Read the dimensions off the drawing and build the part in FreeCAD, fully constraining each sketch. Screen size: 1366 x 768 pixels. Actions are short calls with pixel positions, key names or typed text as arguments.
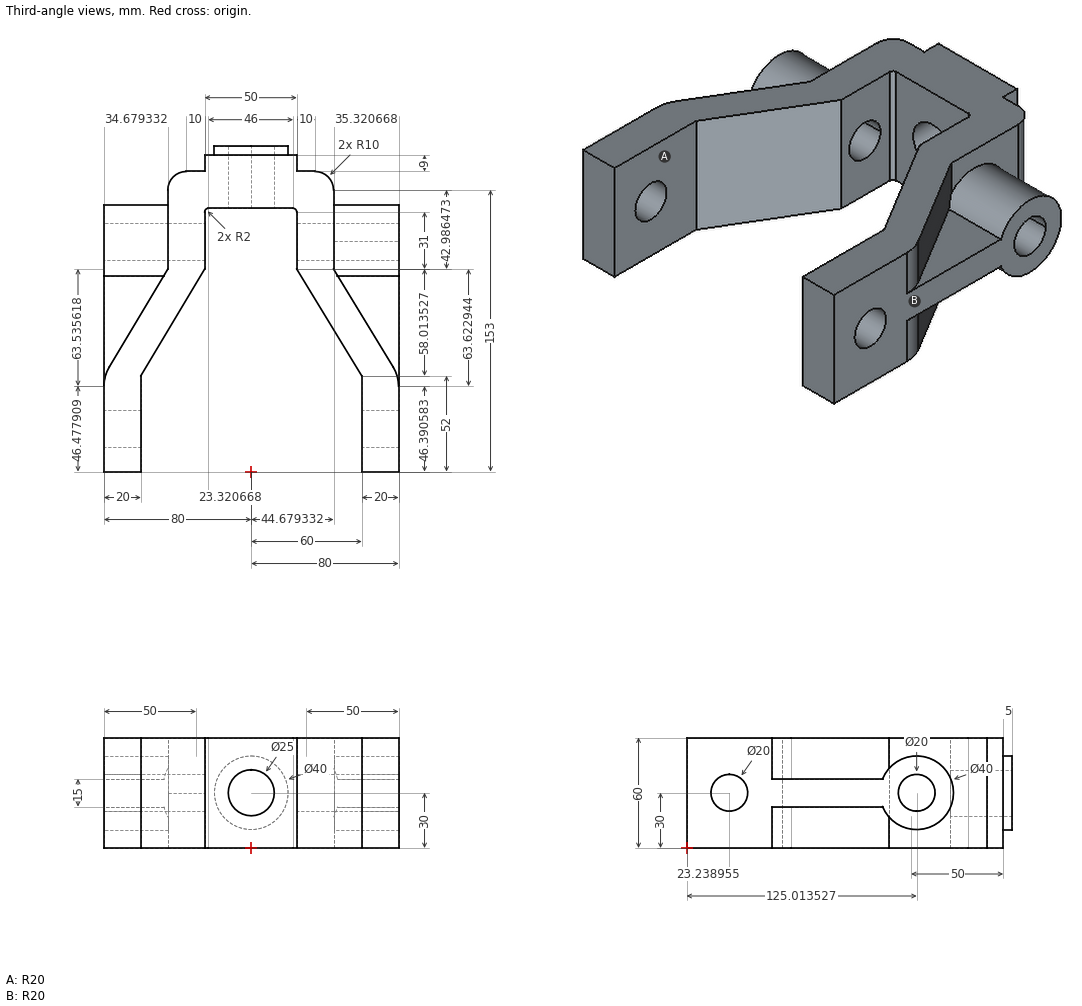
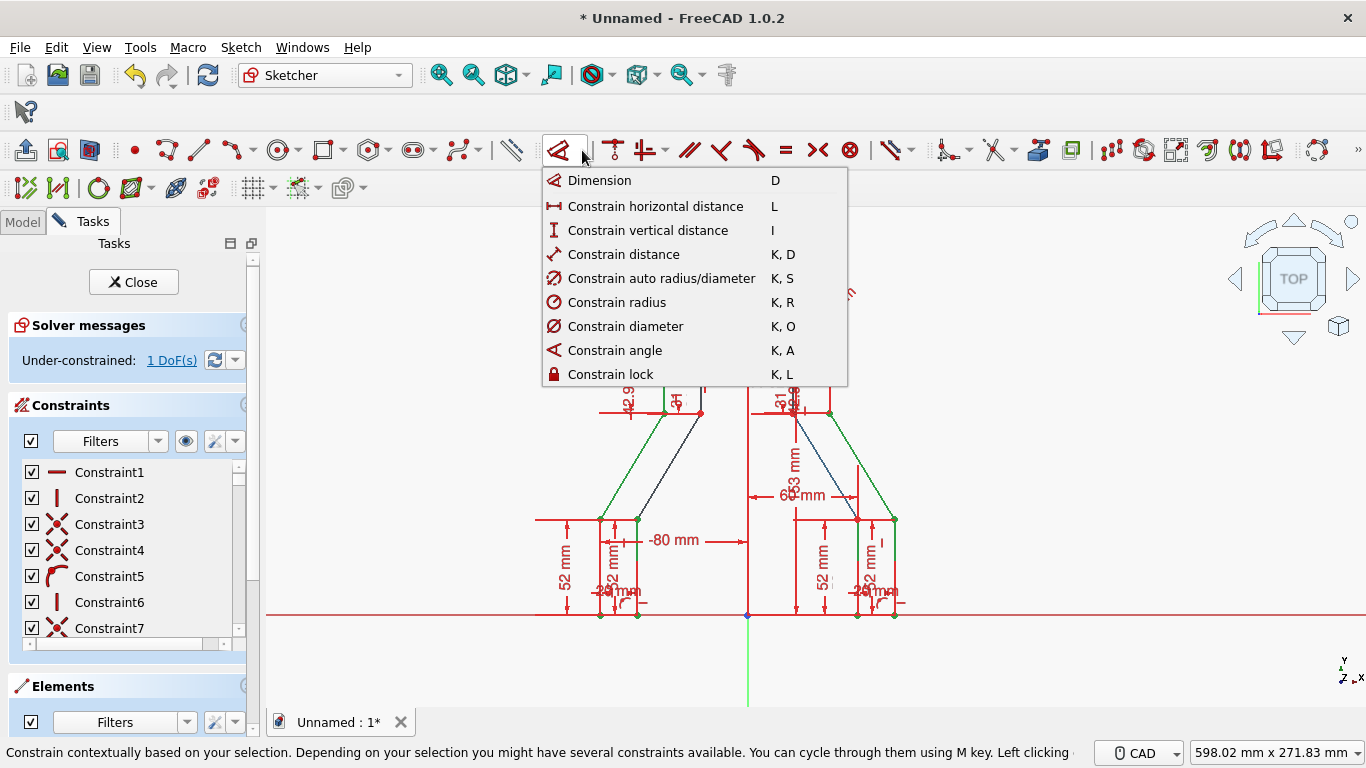
click(695, 230)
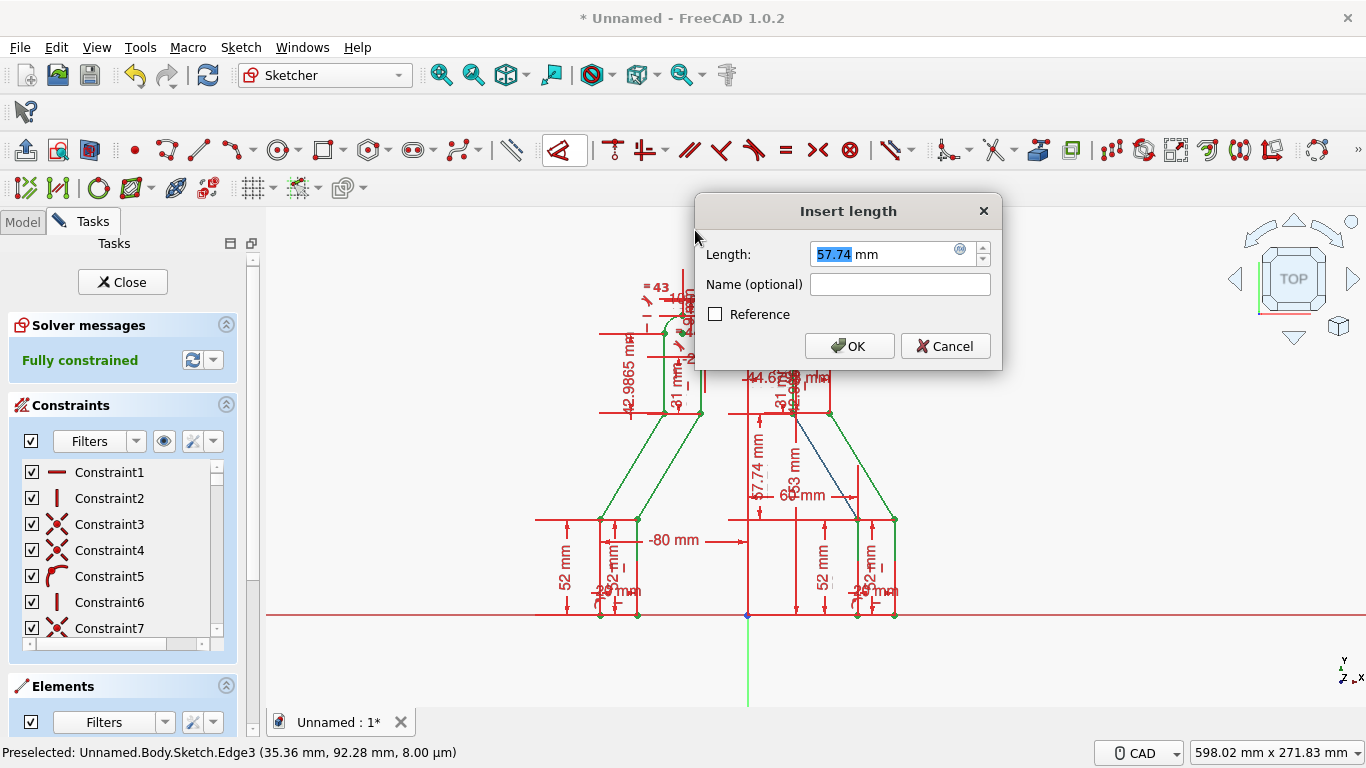
text(58.013527)
key(Return)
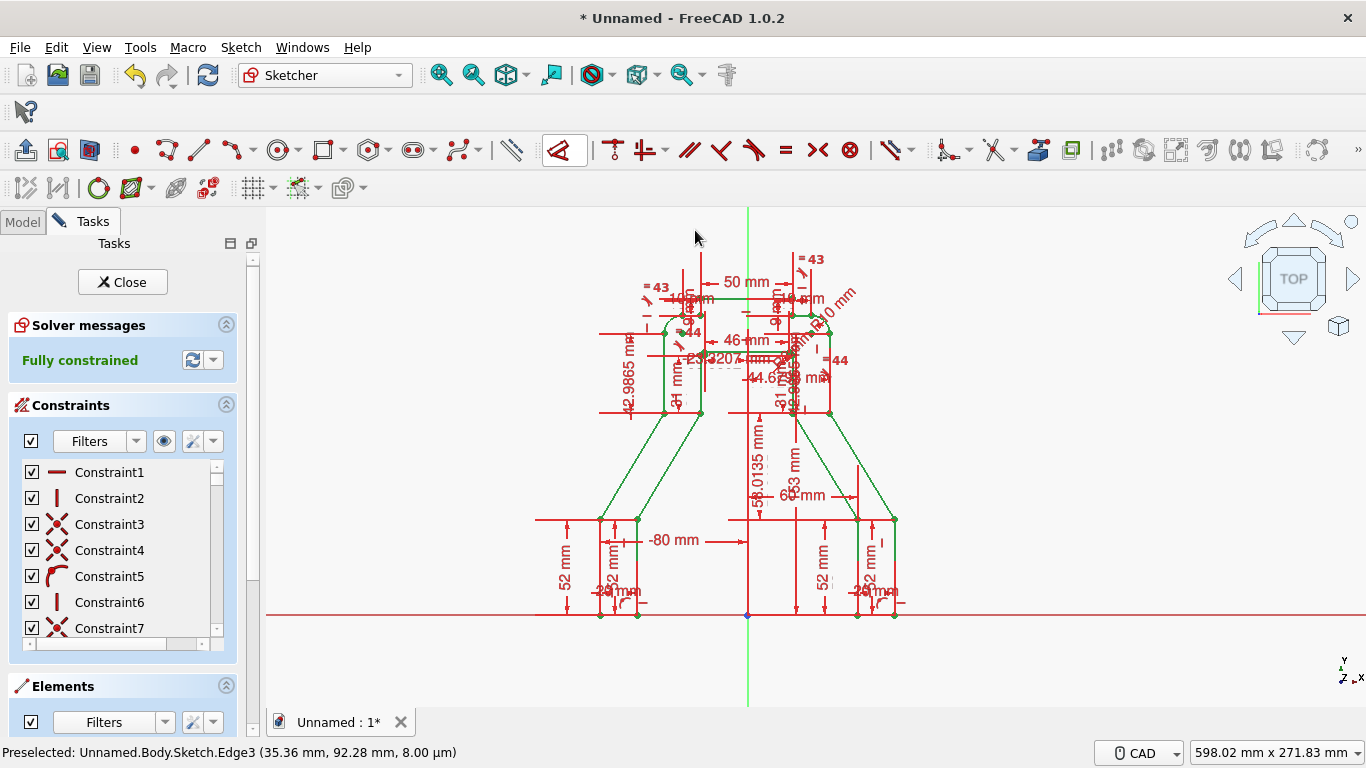
click(123, 282)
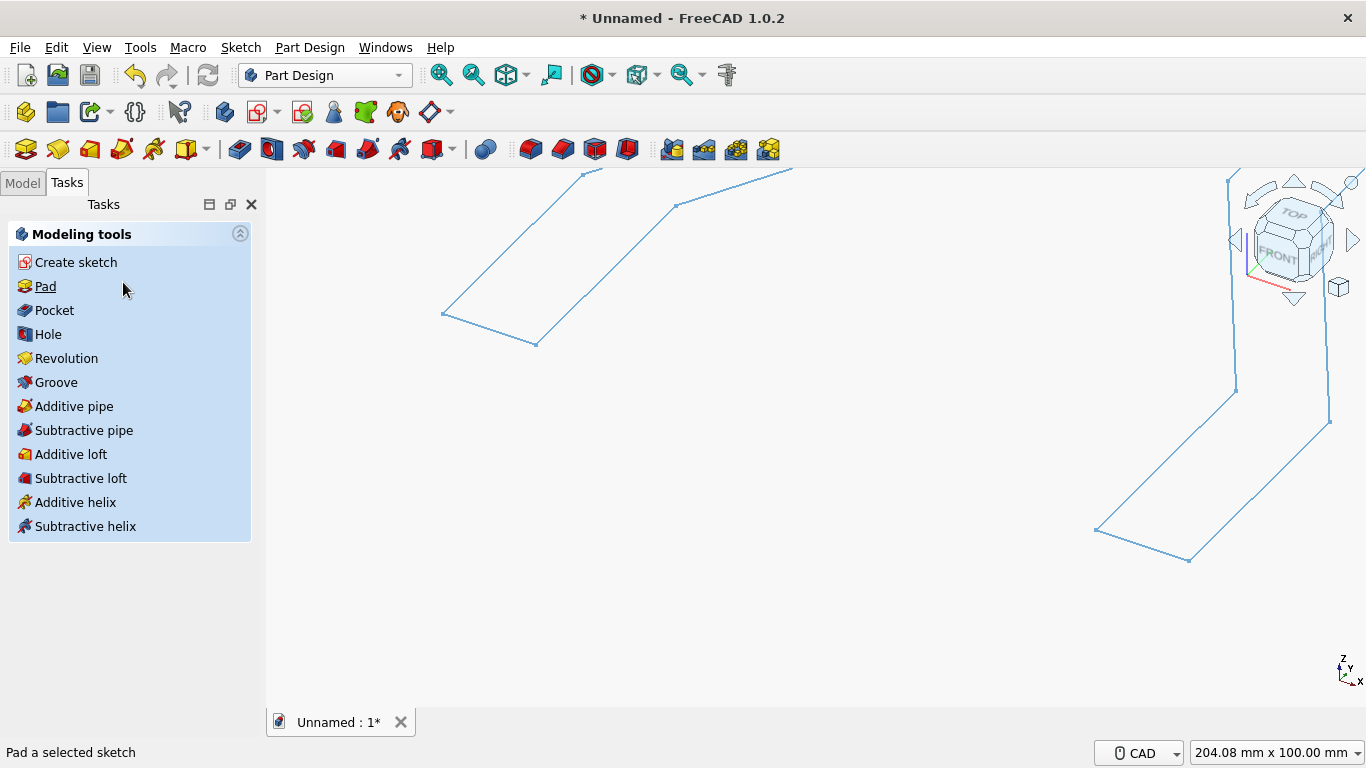
click(26, 150)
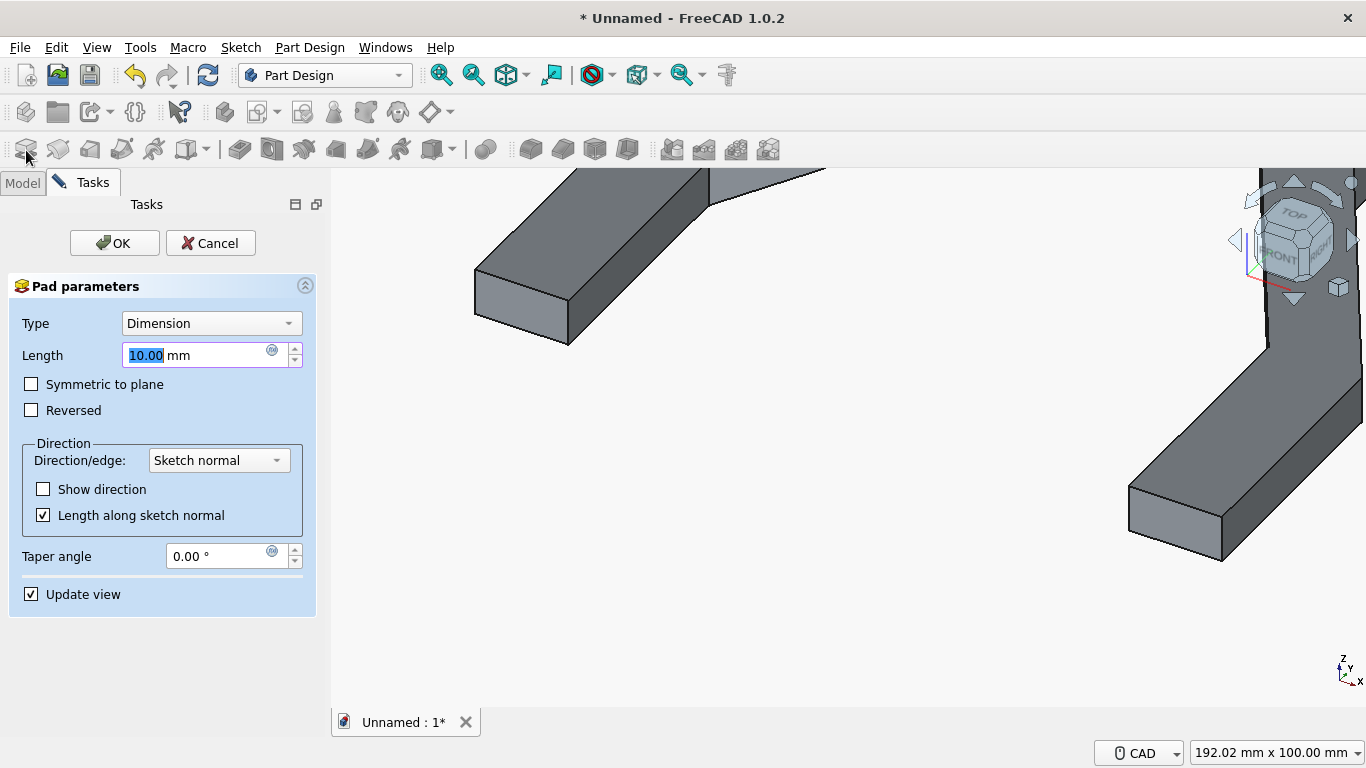
text(60)
key(Tab)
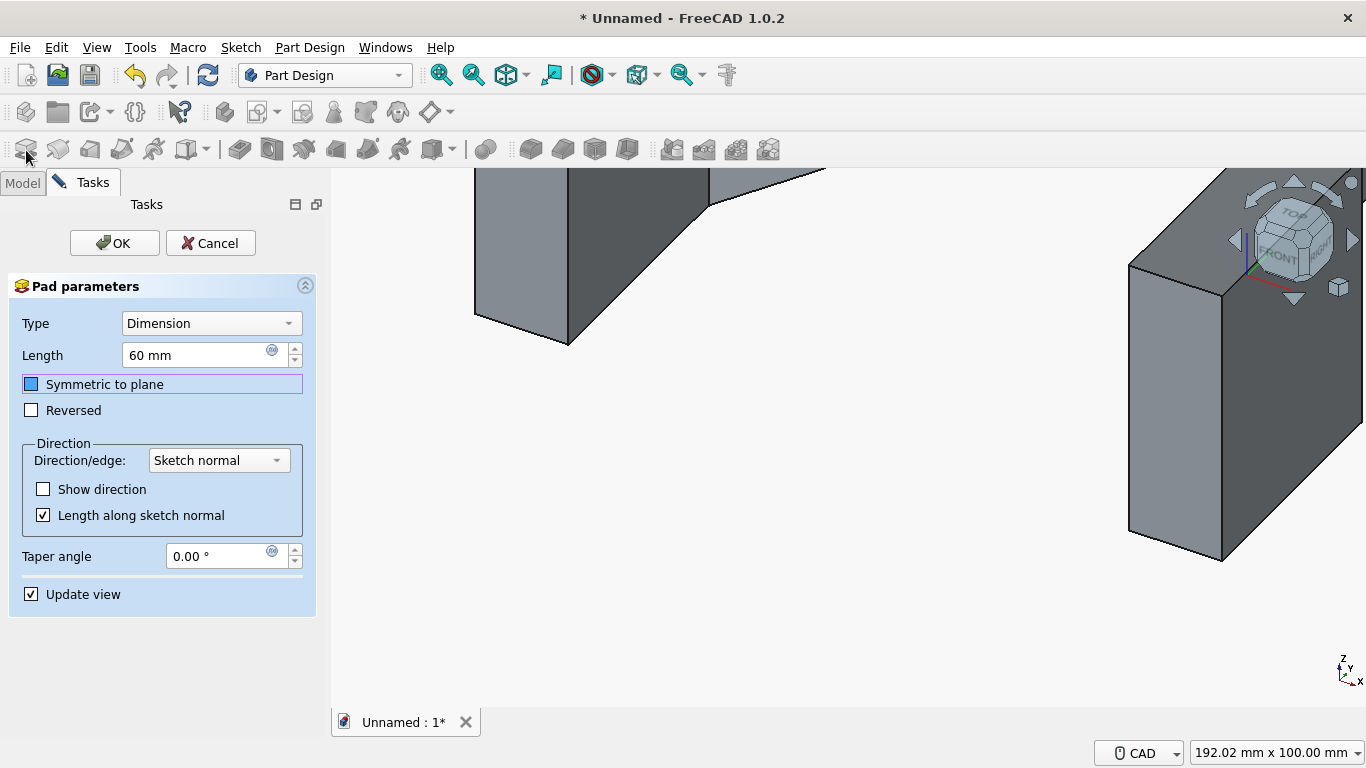
click(115, 243)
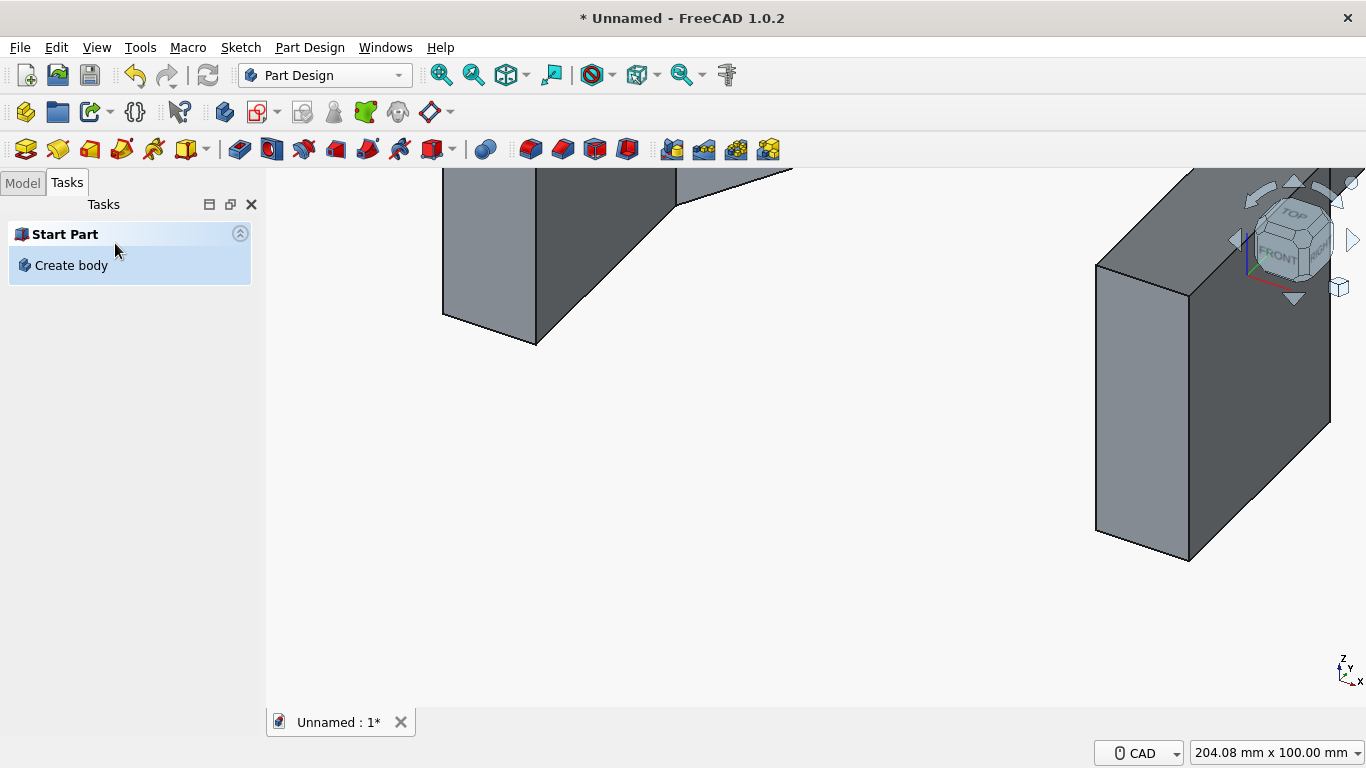
click(442, 76)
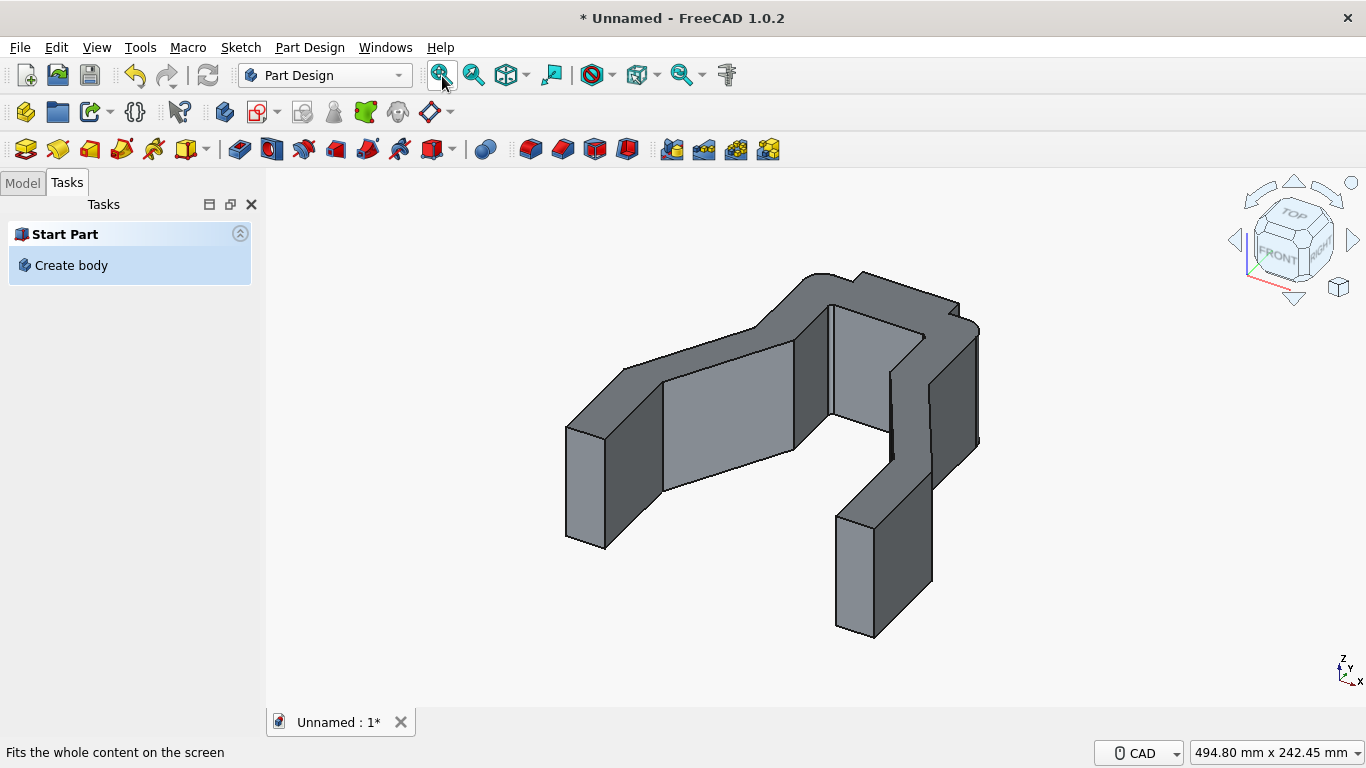
key(4)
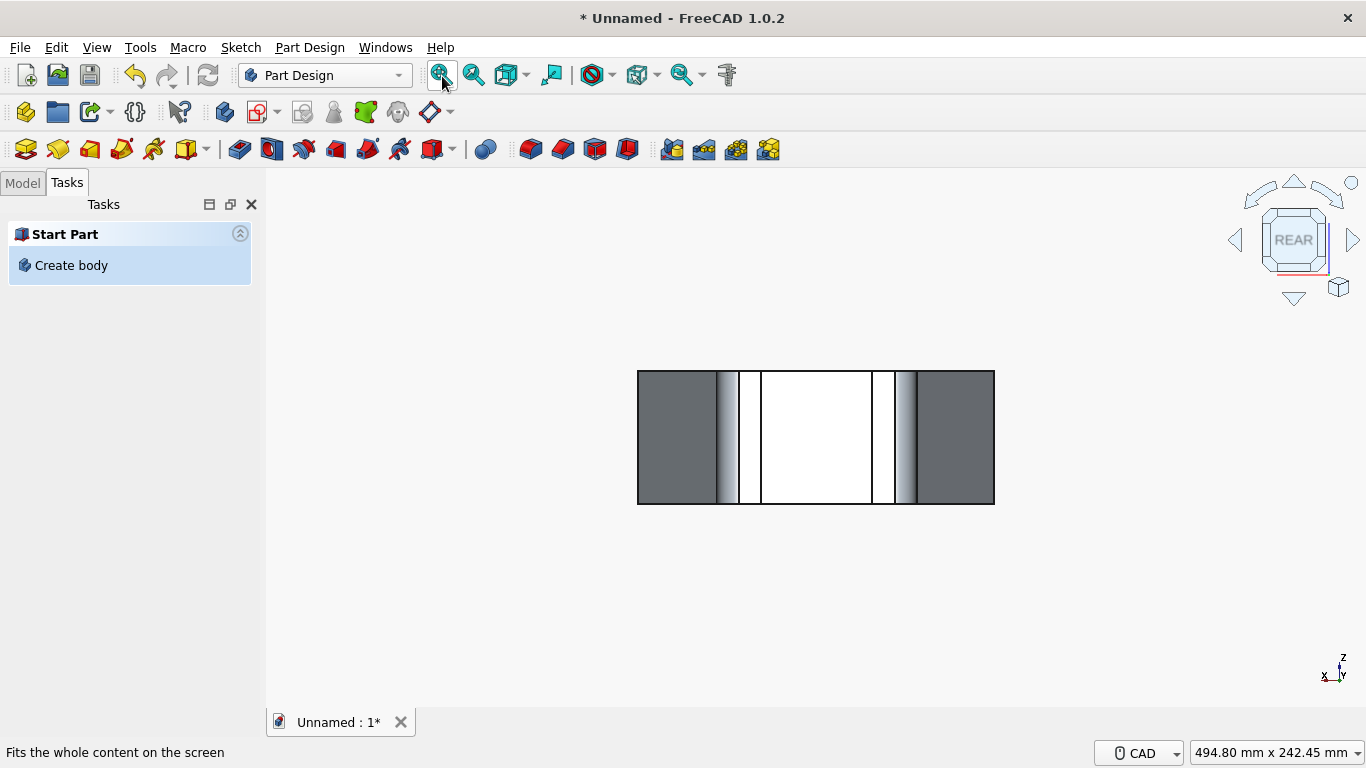
key(v)
key(f)